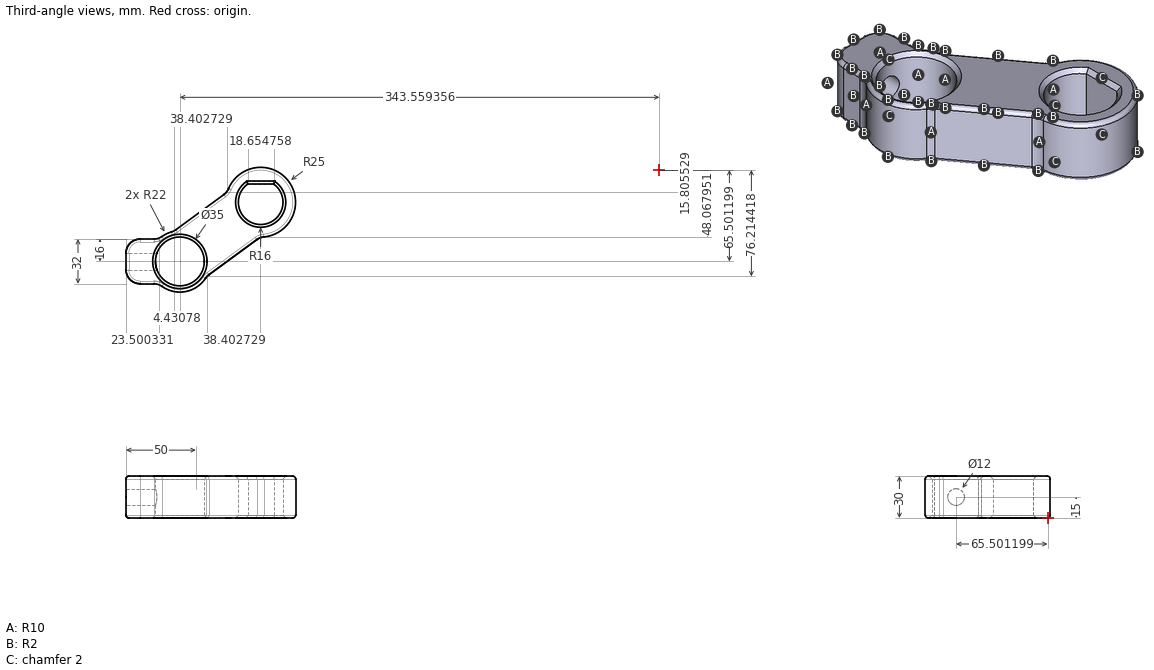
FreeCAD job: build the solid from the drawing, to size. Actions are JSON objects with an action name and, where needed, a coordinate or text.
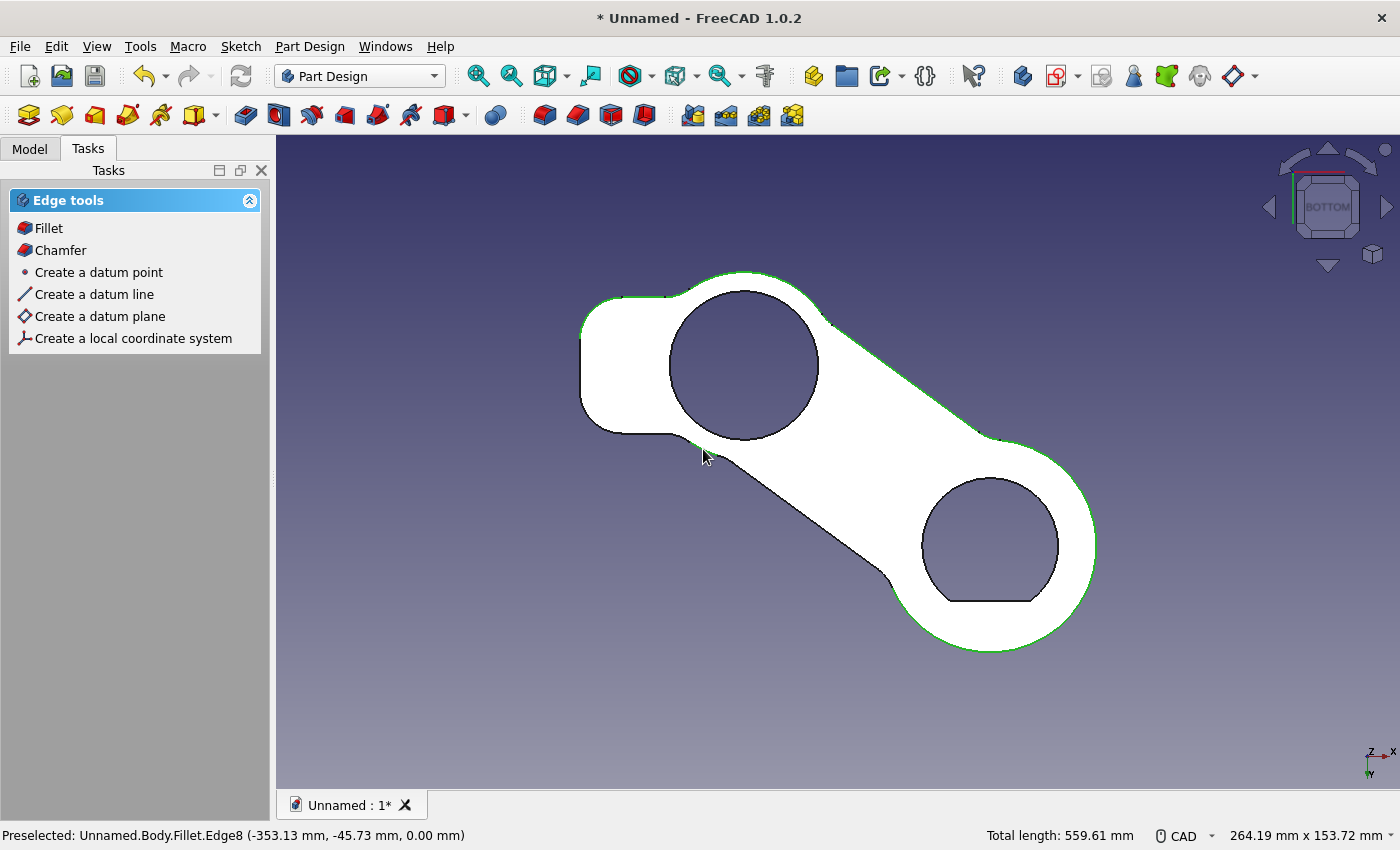
{"action": "left_click", "coordinate": [580, 365], "text": "ctrl"}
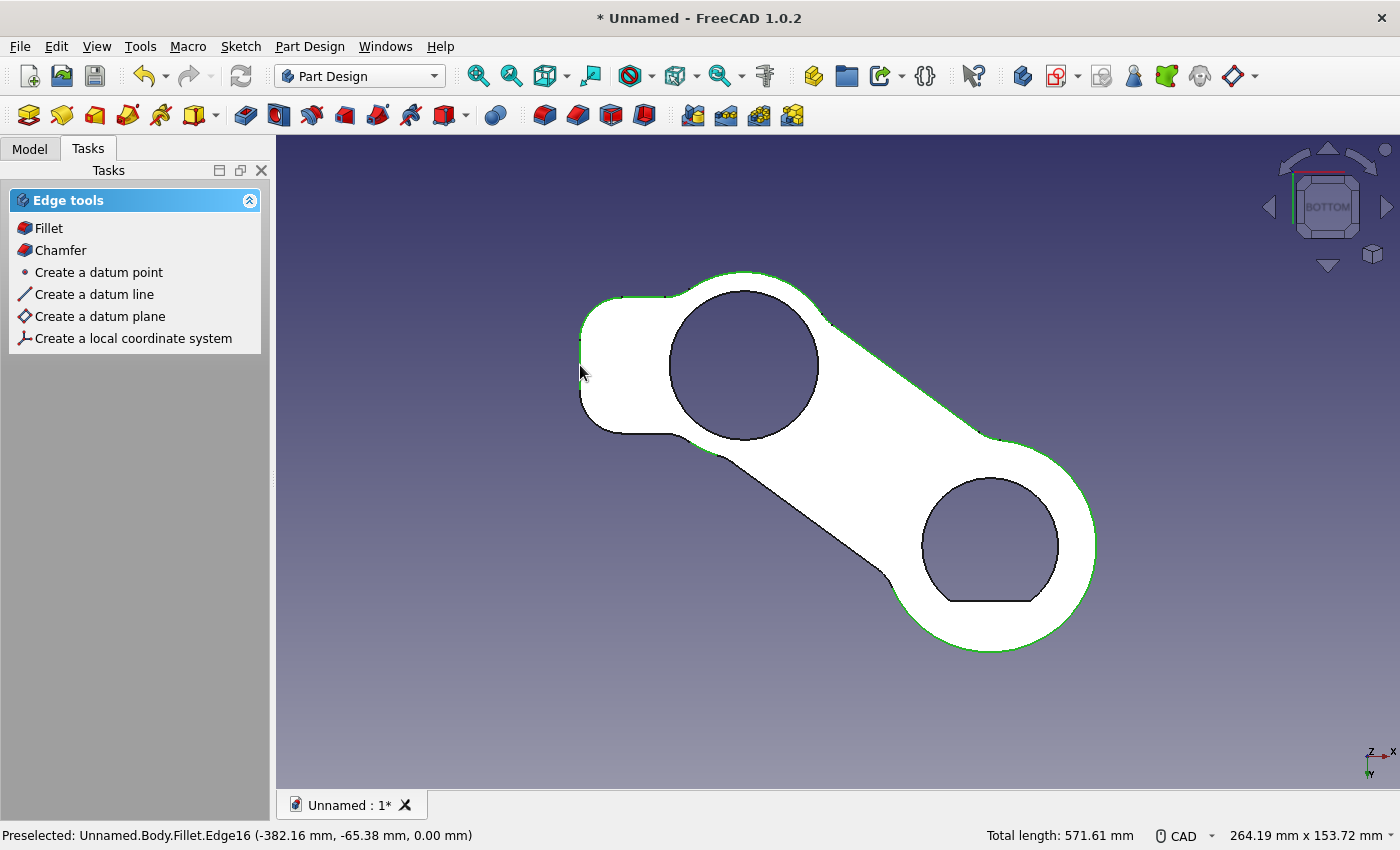
{"action": "left_click", "coordinate": [643, 433], "text": "ctrl"}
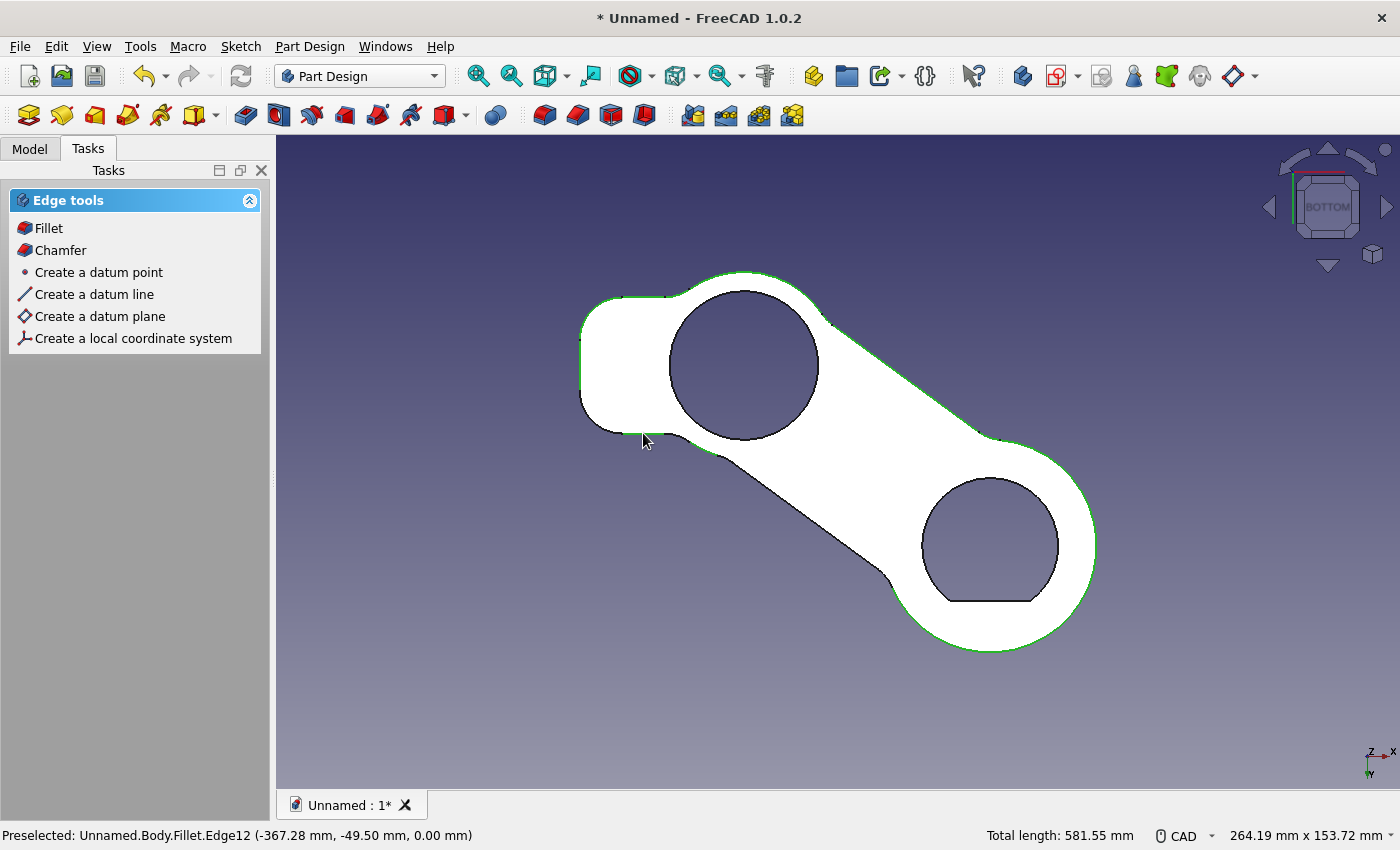
{"action": "left_click", "coordinate": [592, 420], "text": "ctrl"}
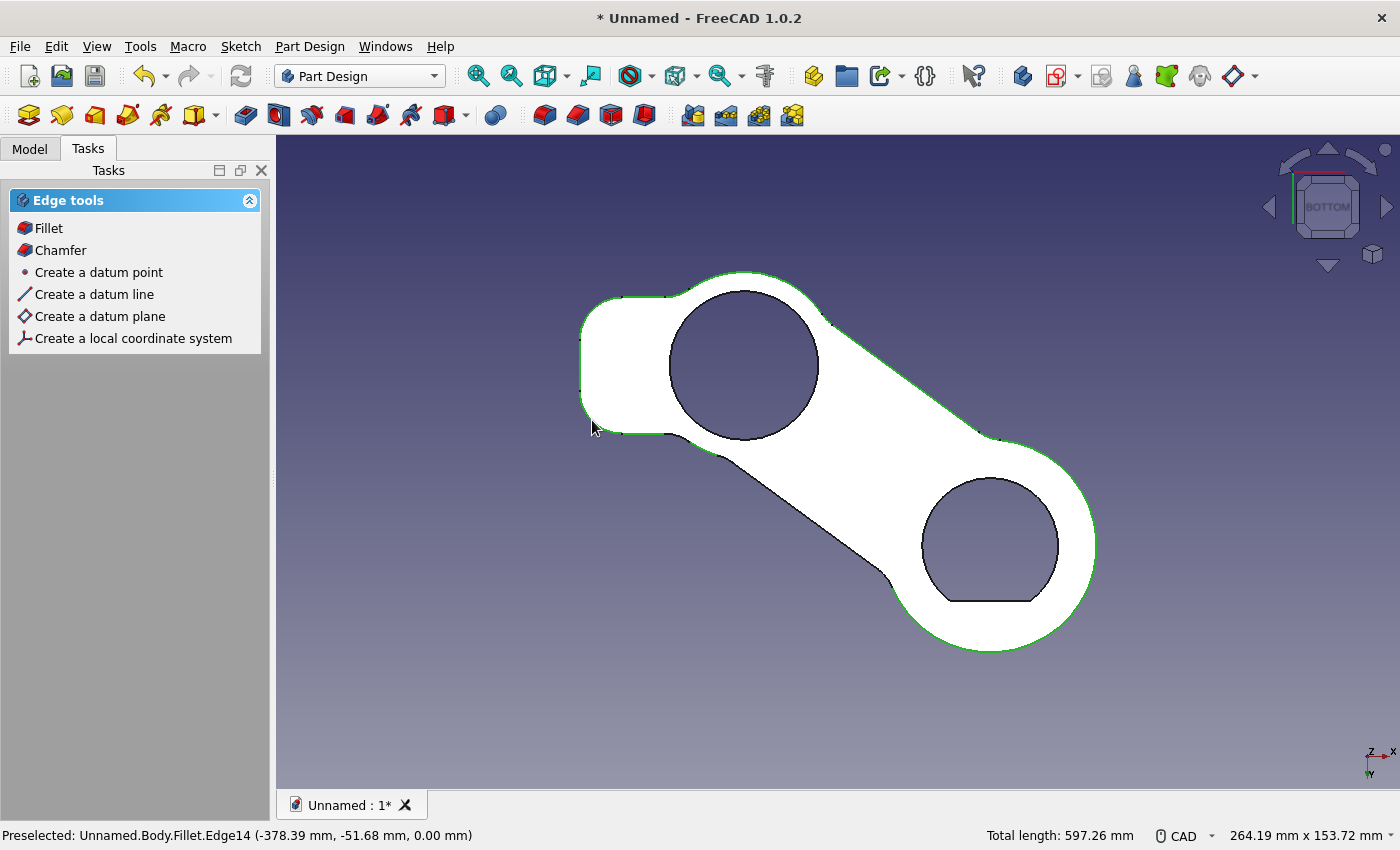
{"action": "left_click", "coordinate": [725, 457], "text": "ctrl"}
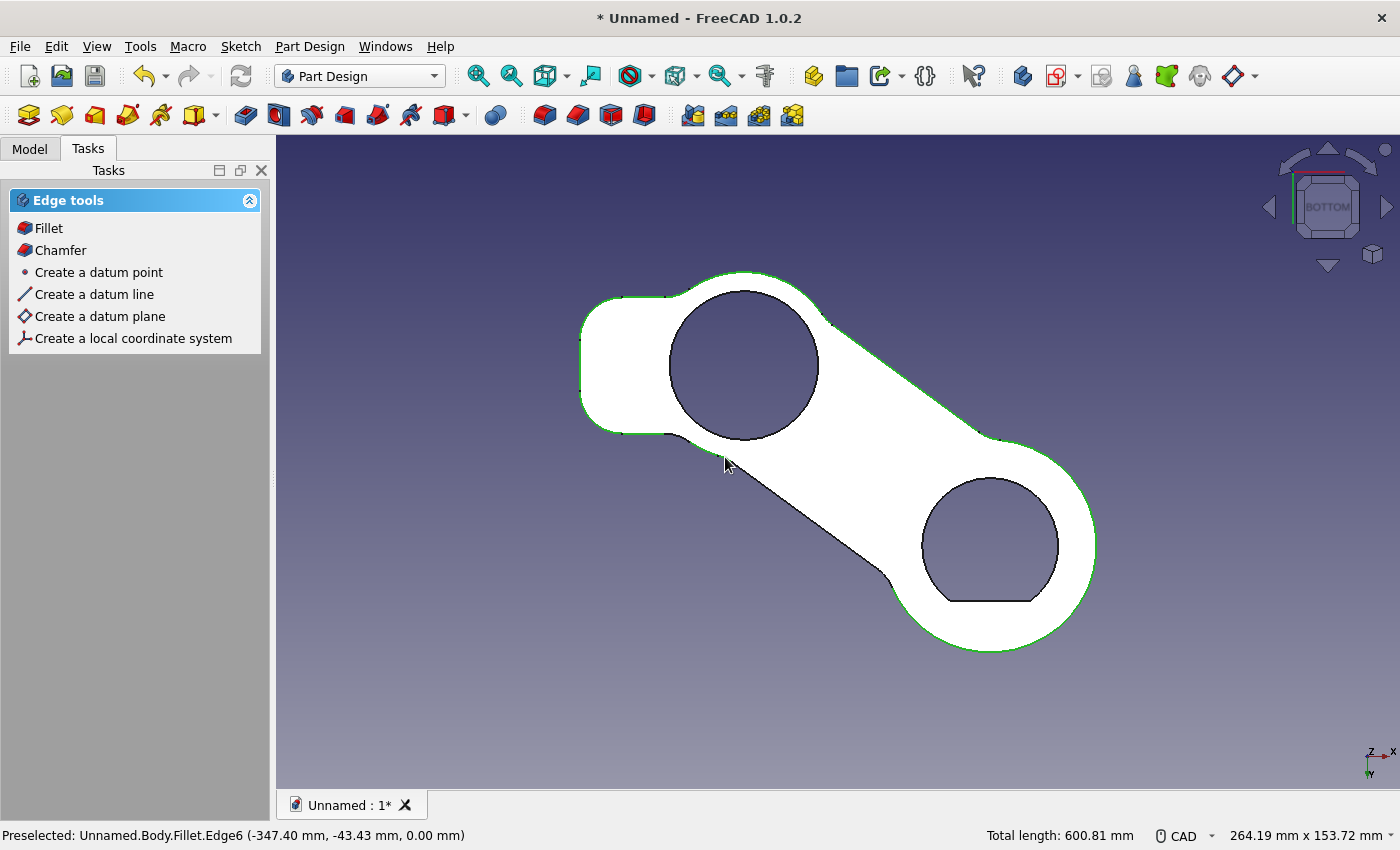
{"action": "left_click", "coordinate": [886, 576], "text": "ctrl"}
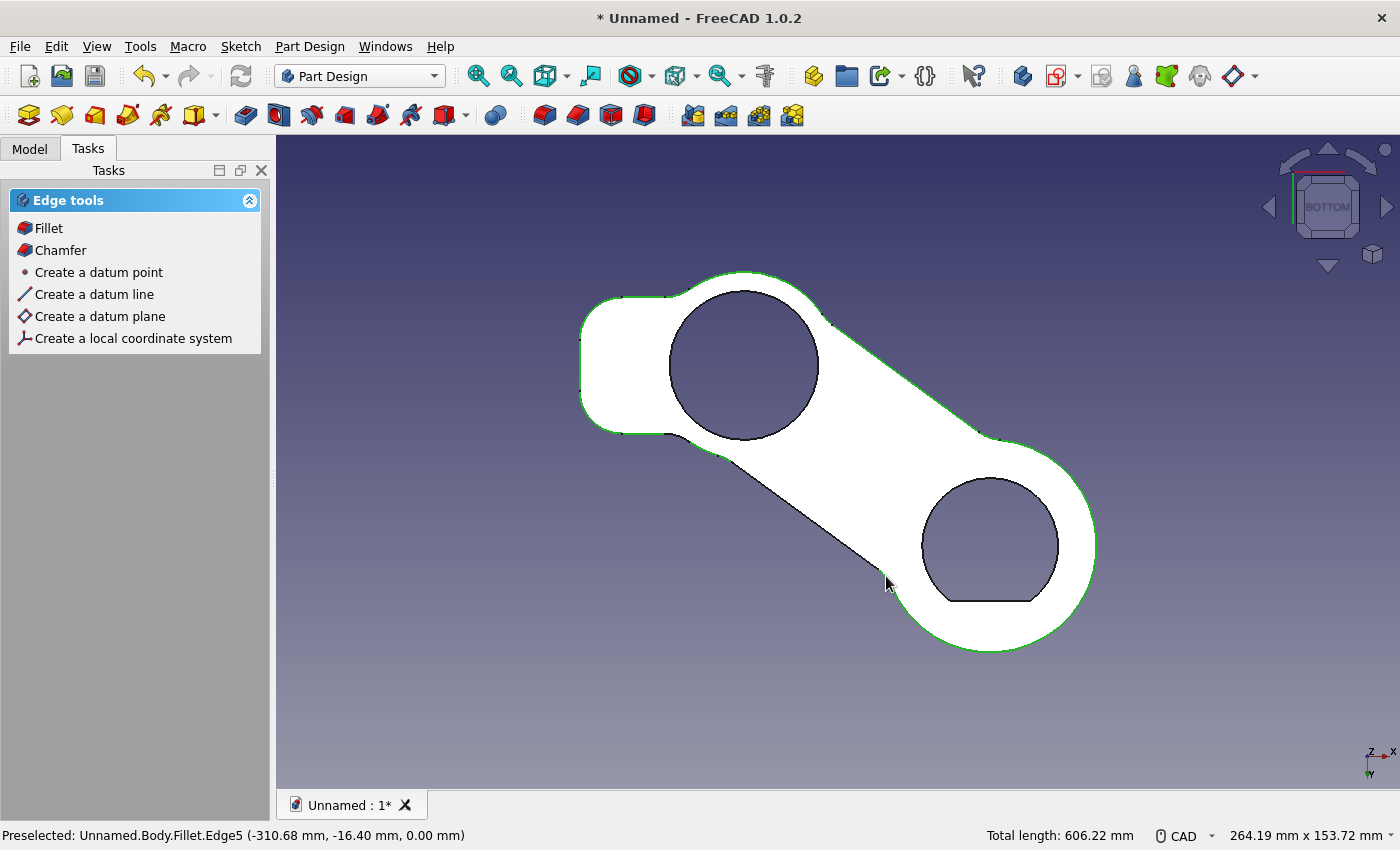
{"action": "left_click", "coordinate": [682, 437], "text": "ctrl"}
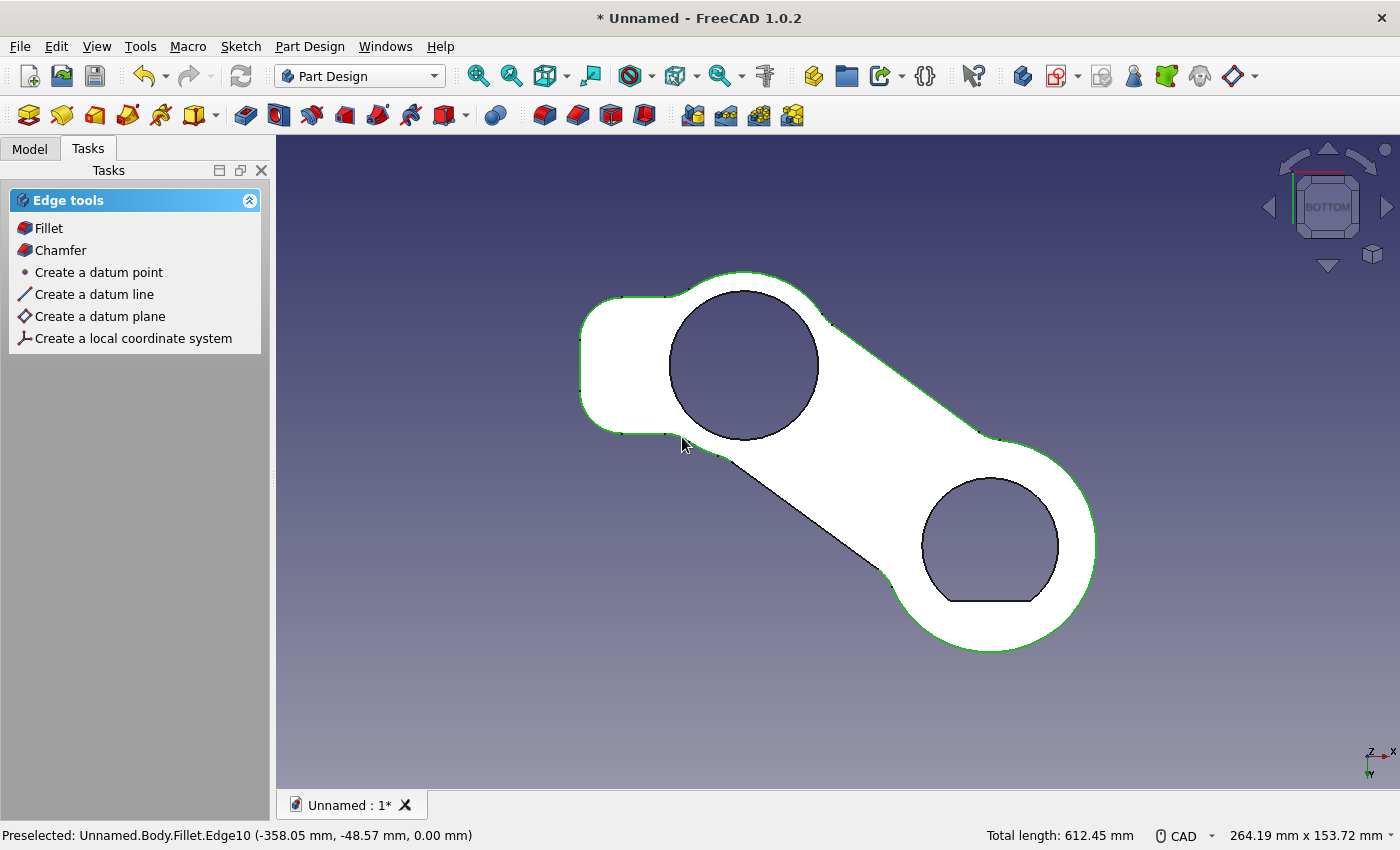
{"action": "key", "text": "4"}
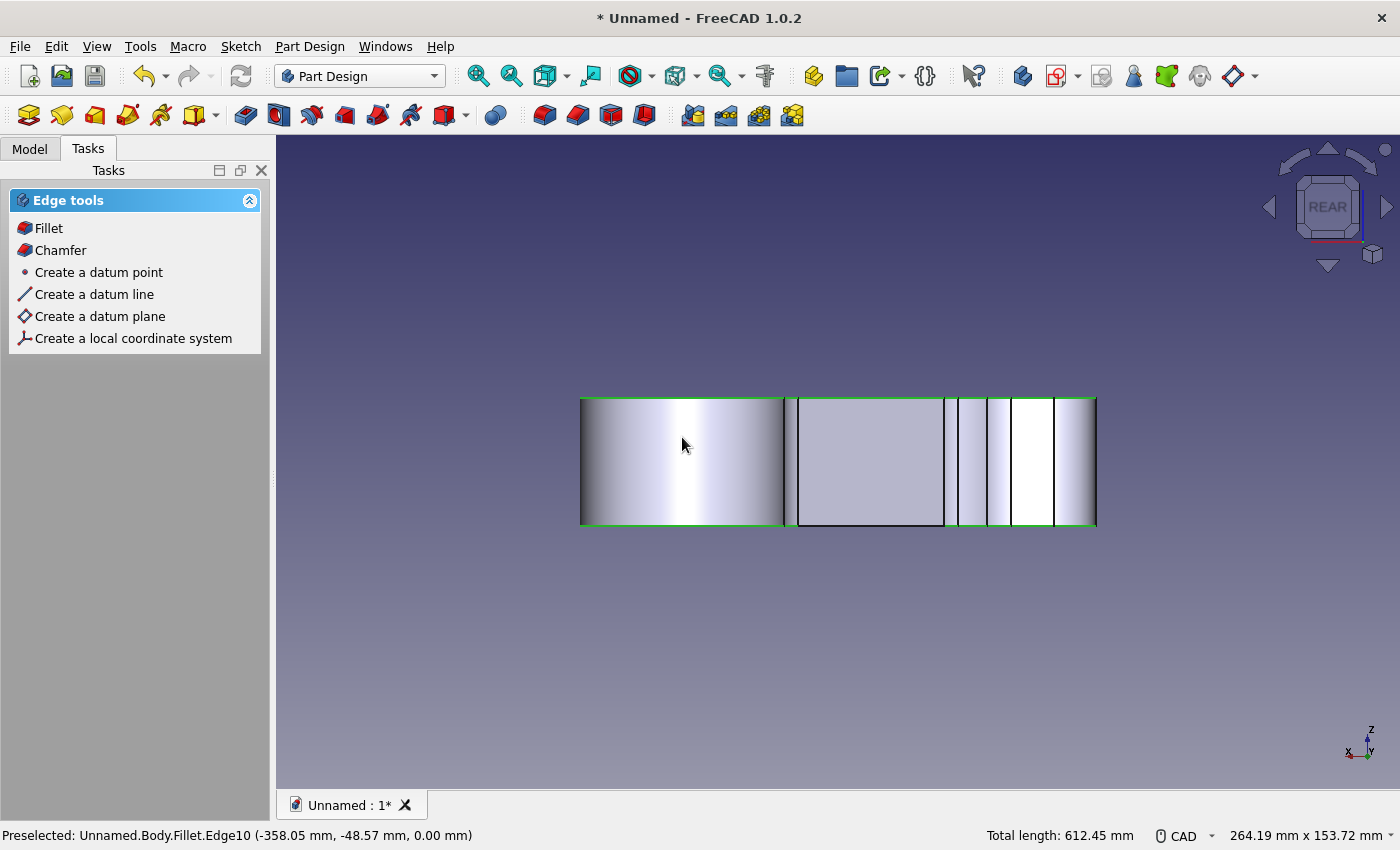
{"action": "left_click", "coordinate": [871, 525], "text": "ctrl"}